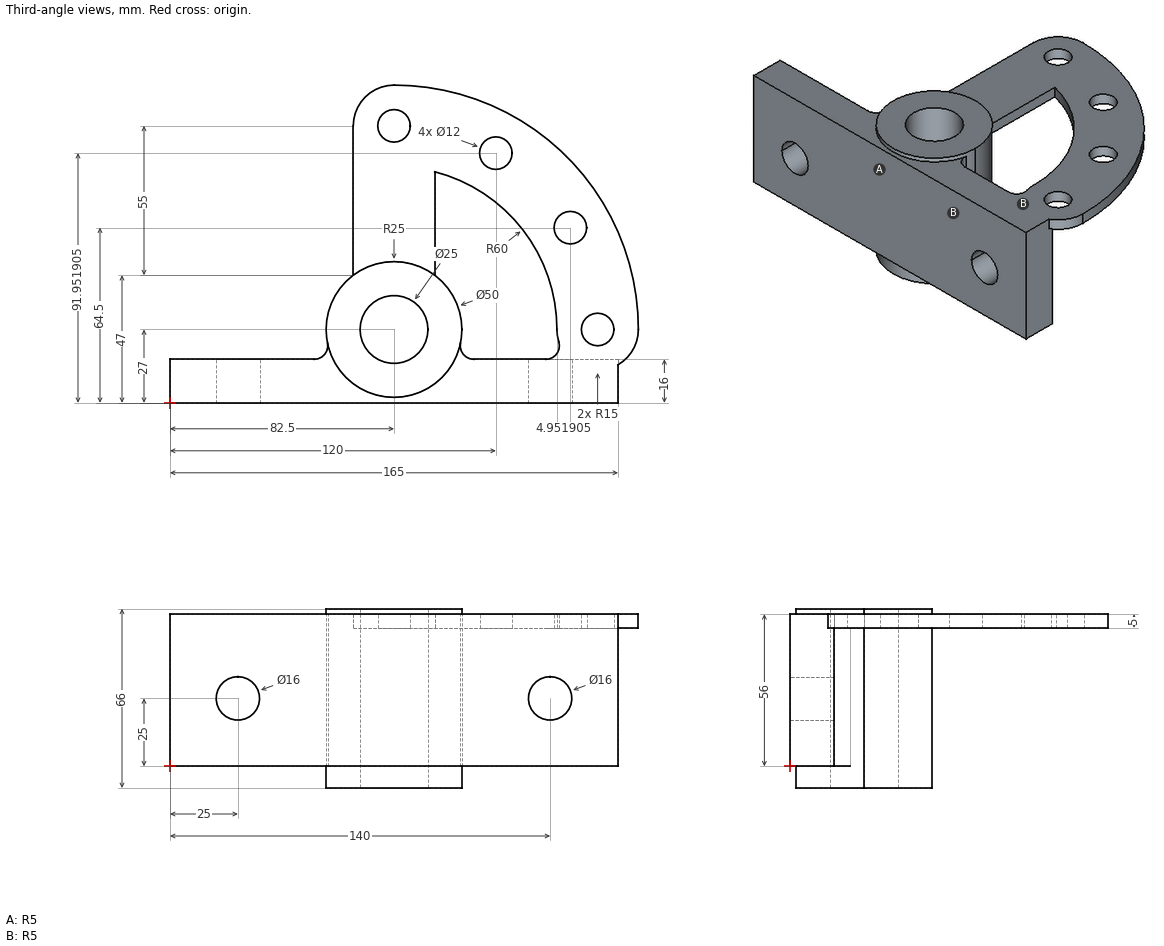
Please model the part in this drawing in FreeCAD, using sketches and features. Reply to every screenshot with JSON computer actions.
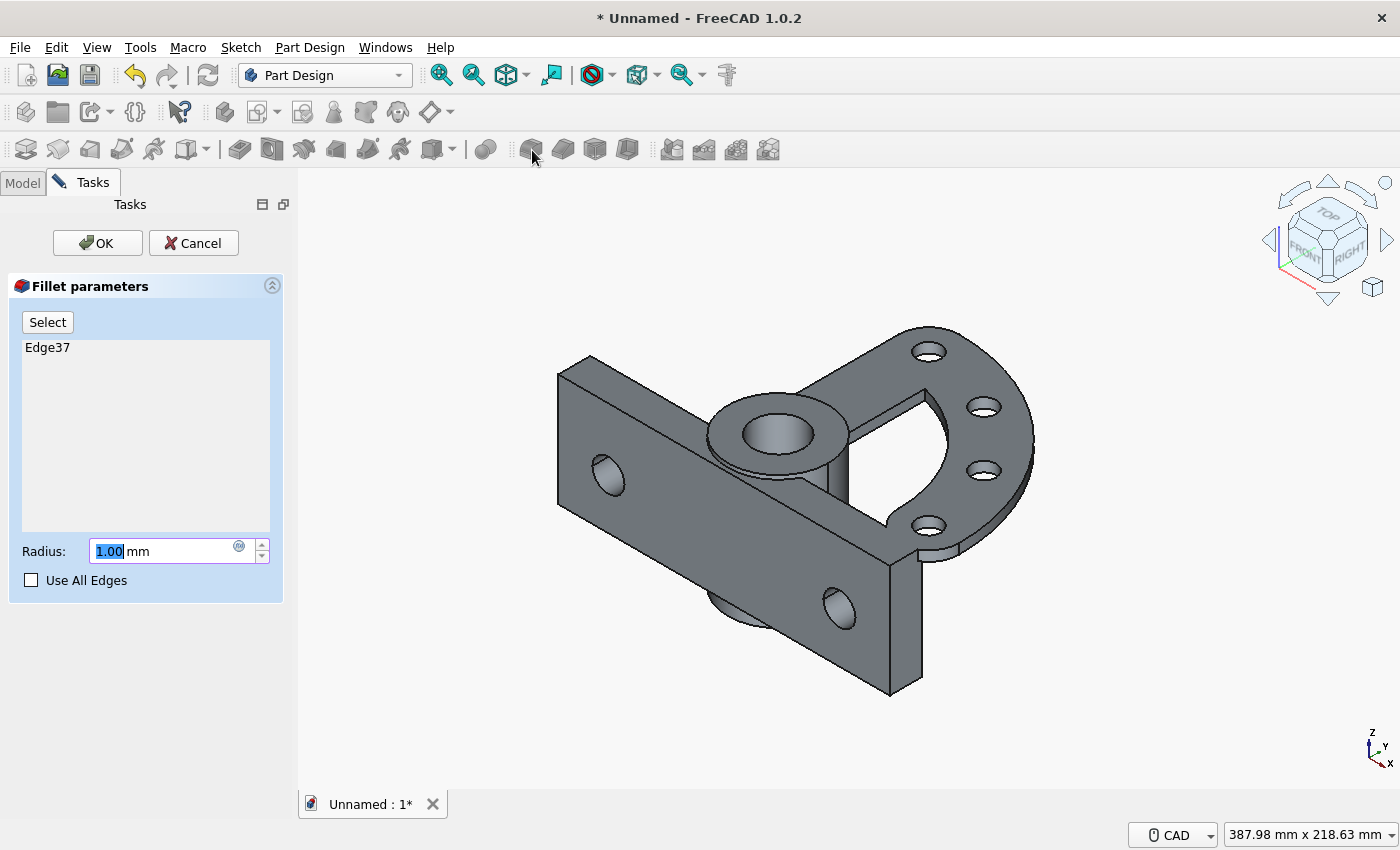
{"action": "type", "text": "5"}
{"action": "key", "text": "Tab"}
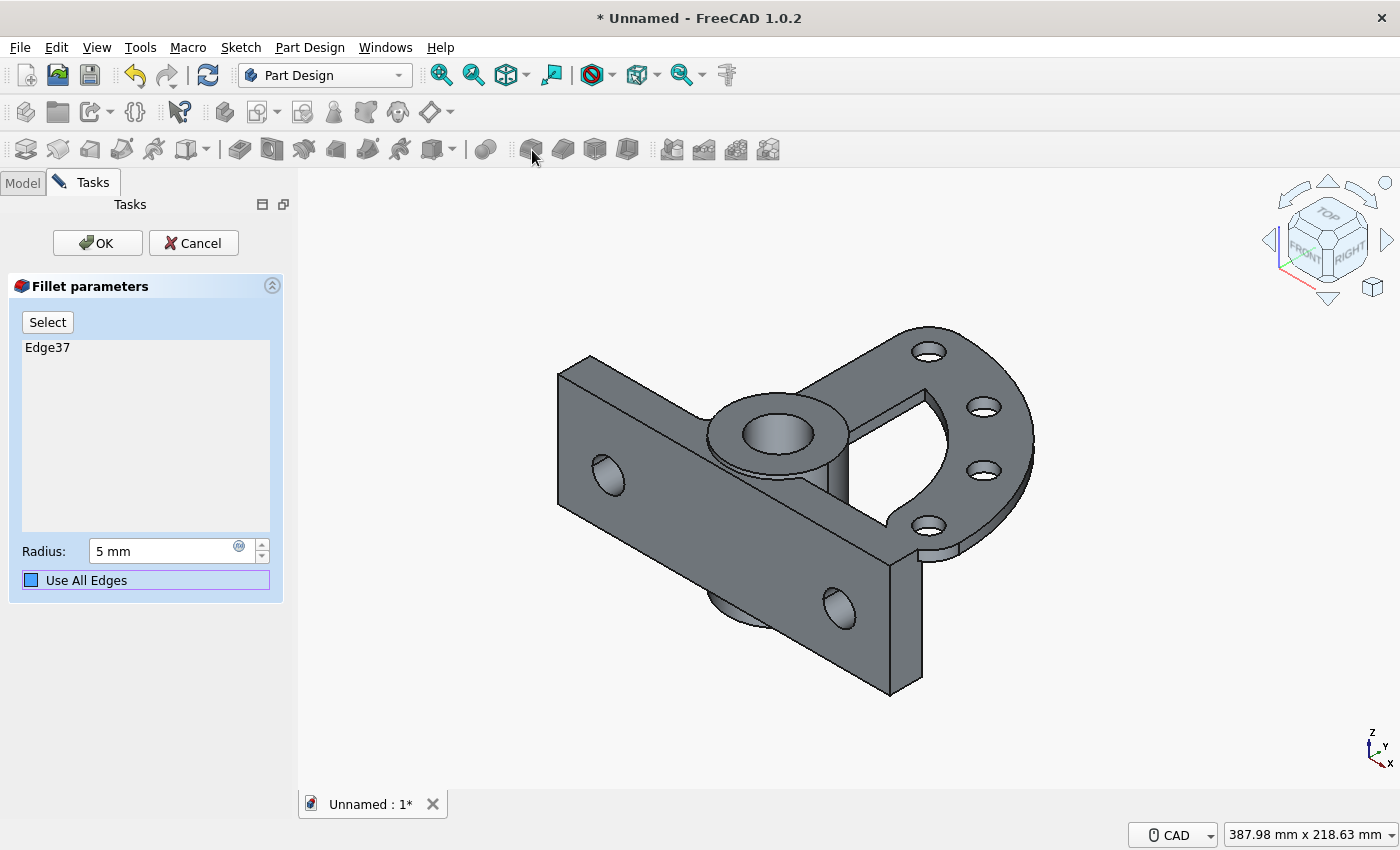
{"action": "left_click", "coordinate": [98, 243]}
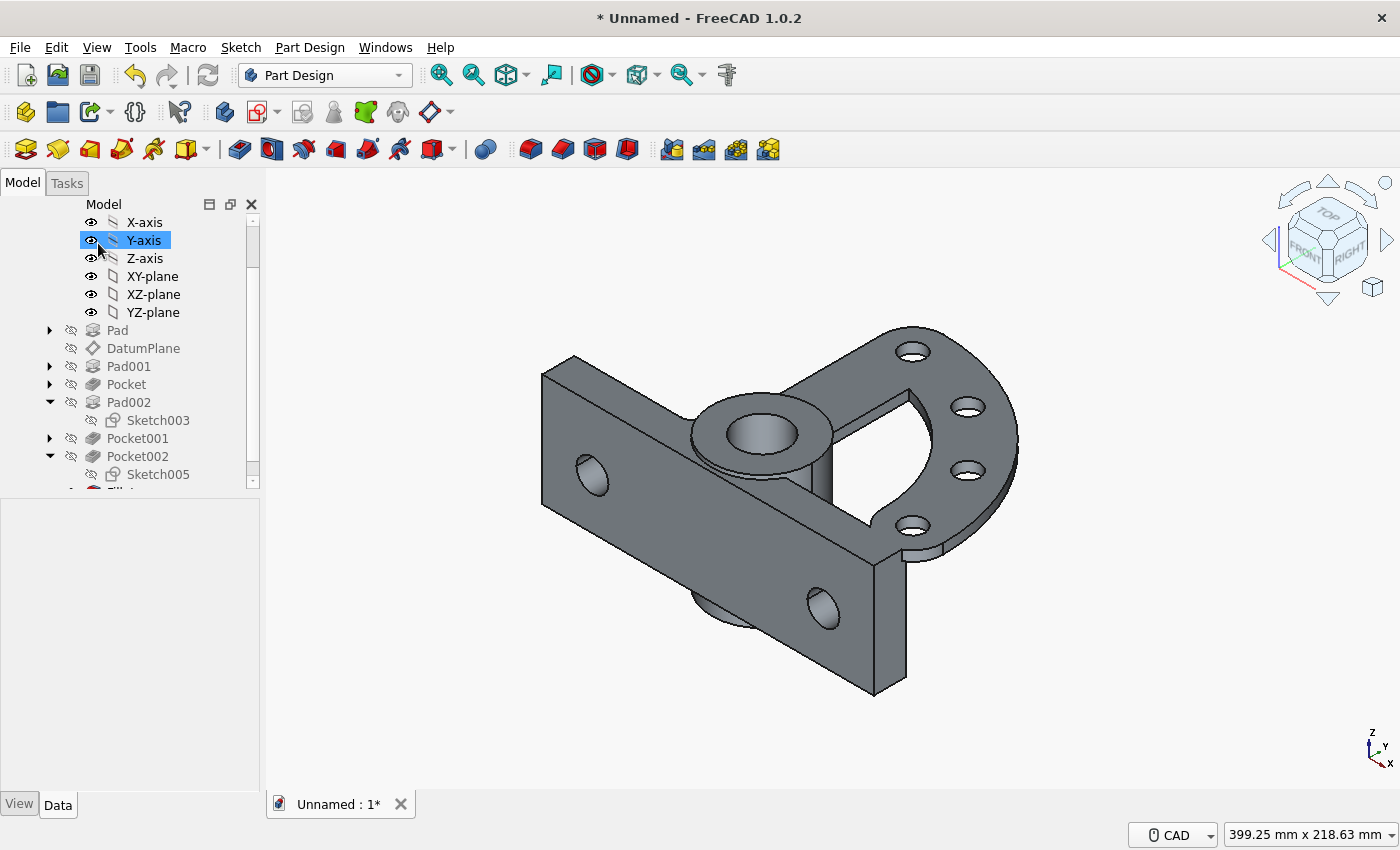
{"action": "key", "text": "2"}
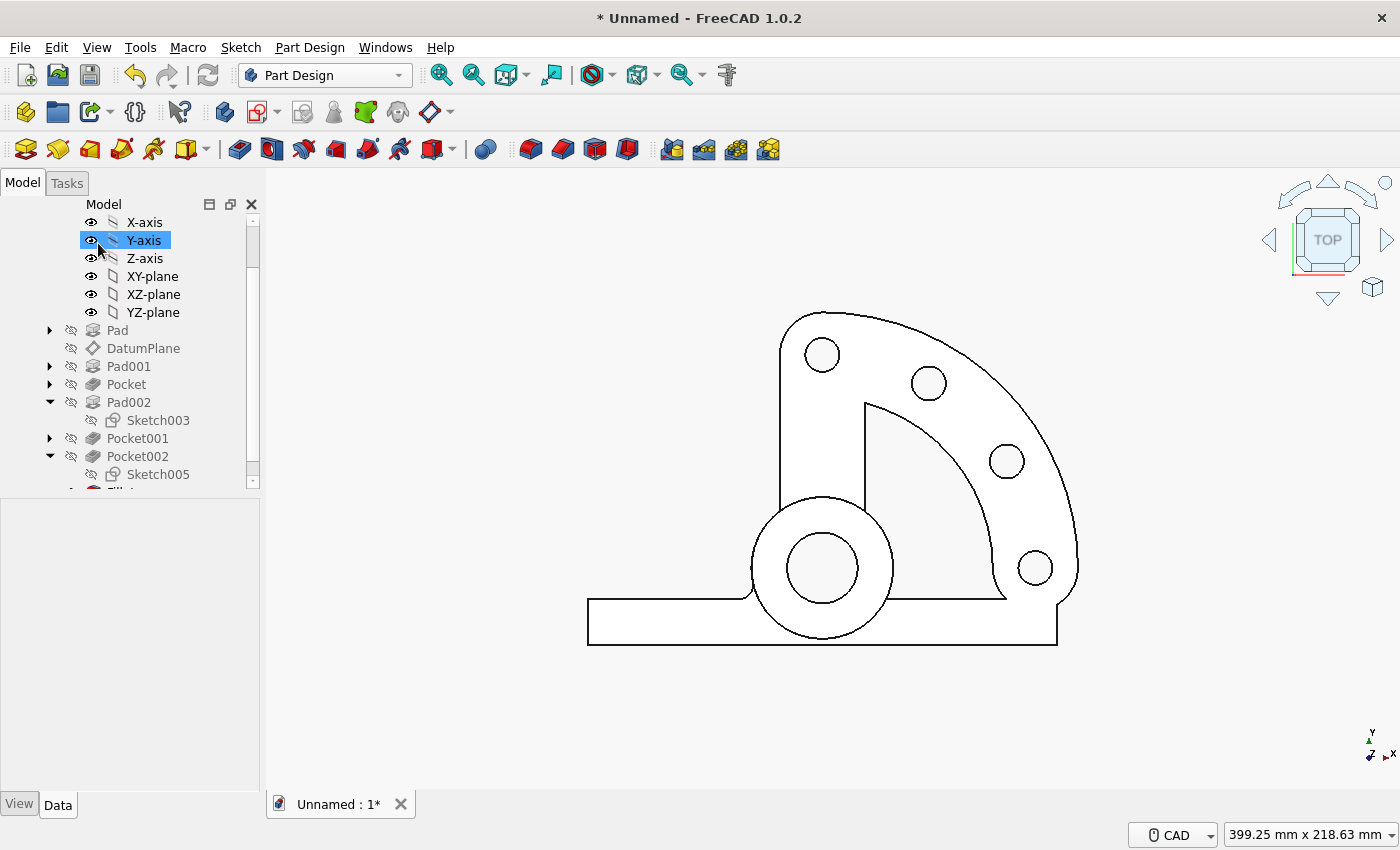
{"action": "key", "text": "0"}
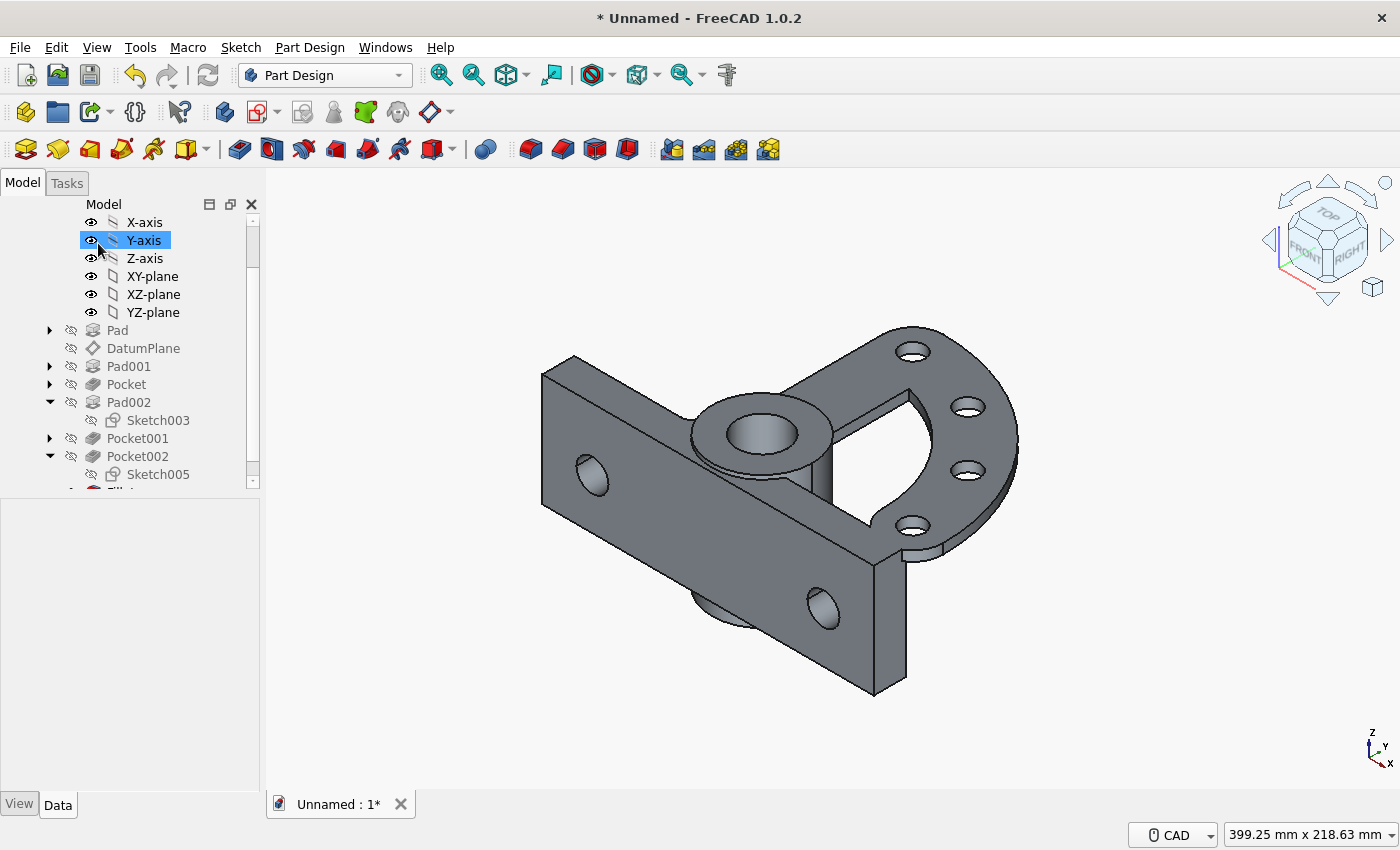
{"action": "key", "text": "1"}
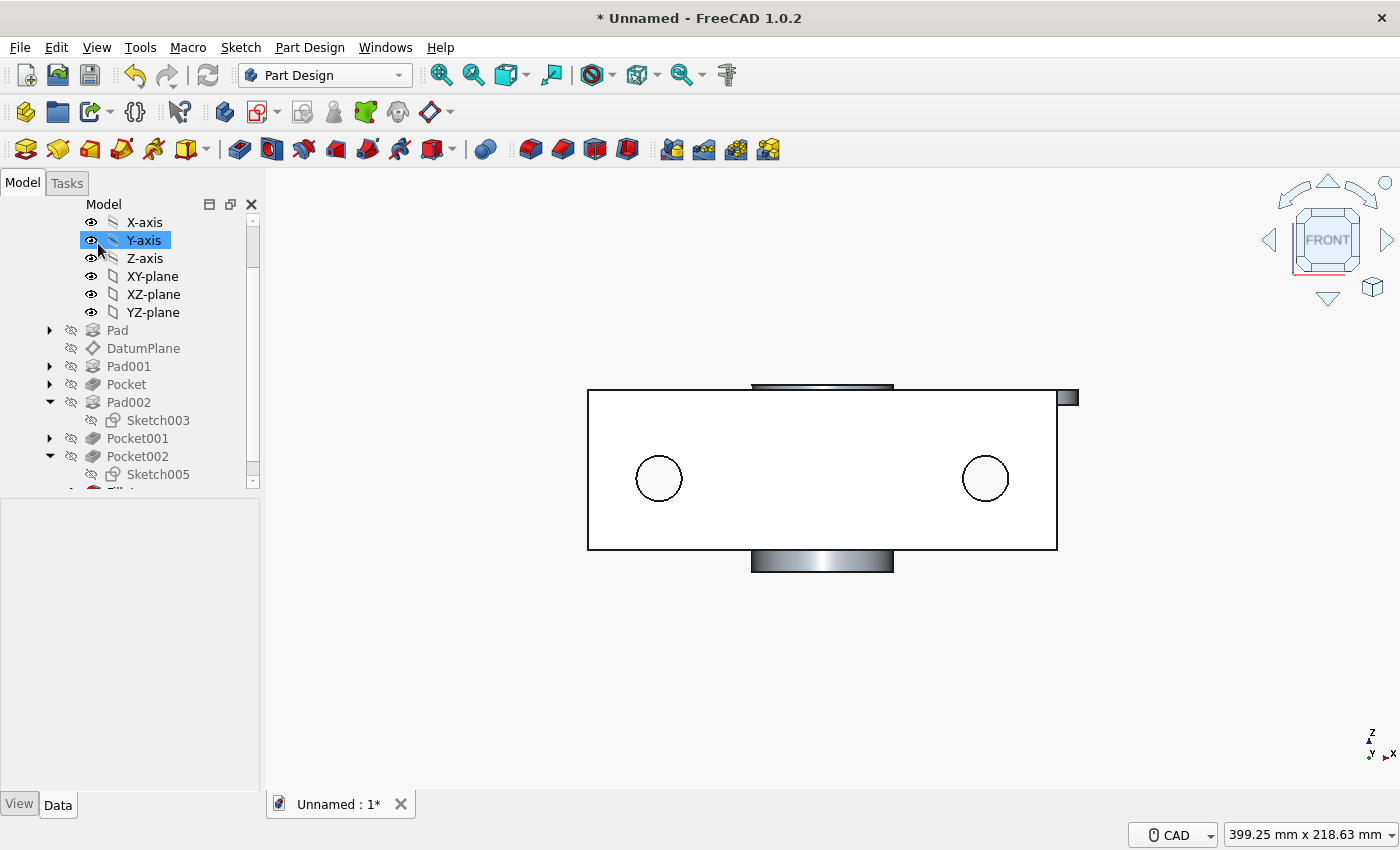
{"action": "key", "text": "v f"}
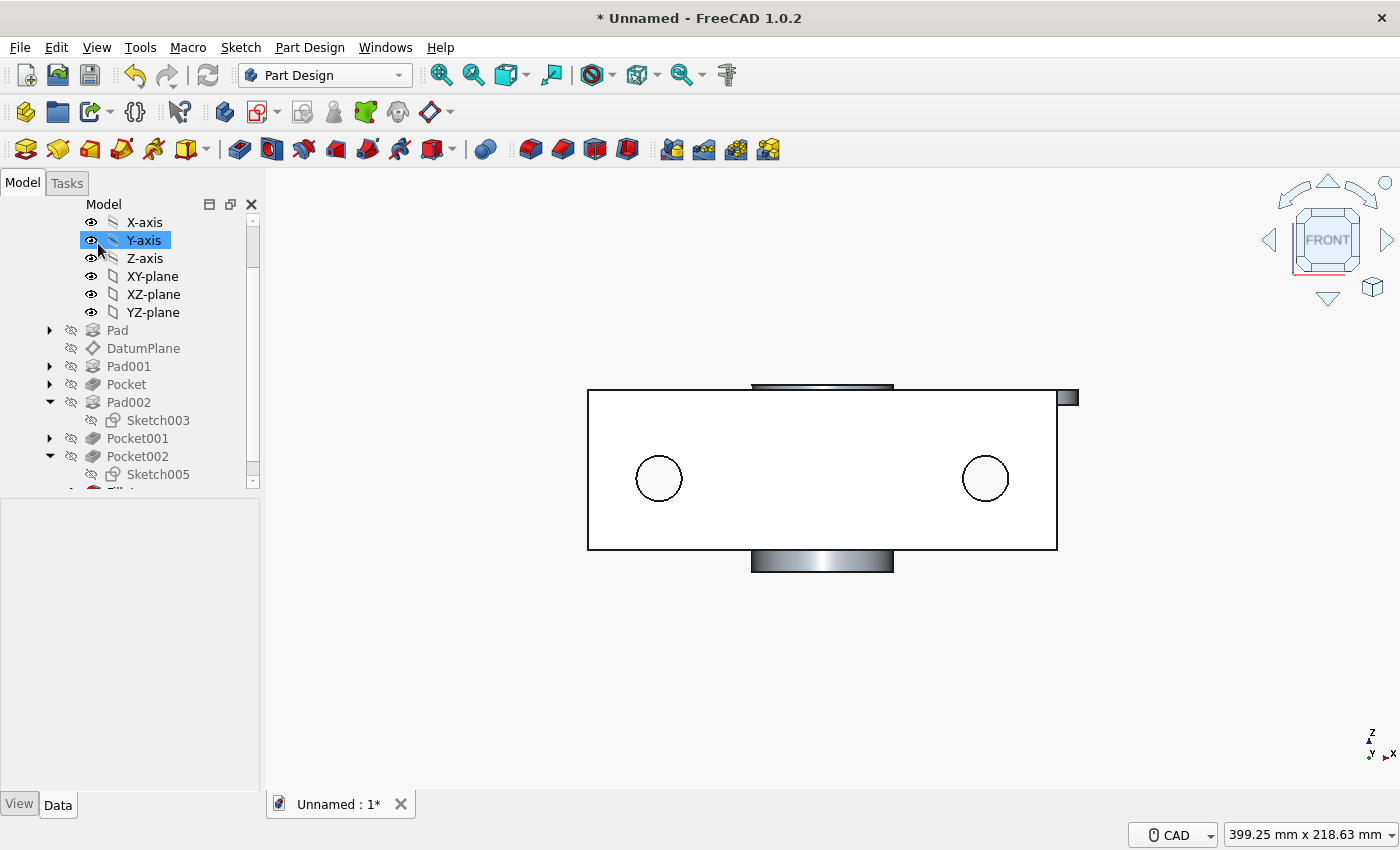
{"action": "key", "text": "3"}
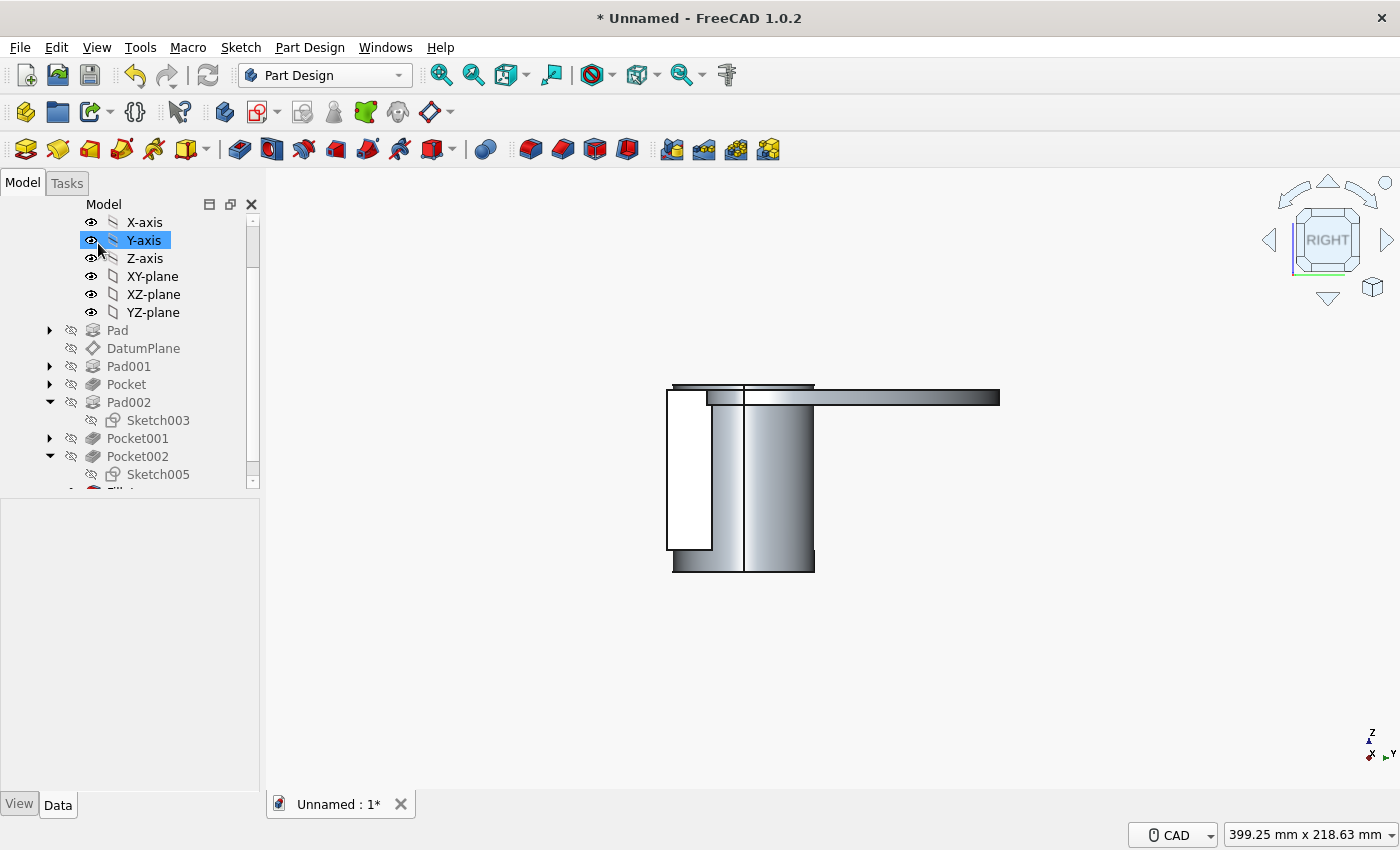
{"action": "key", "text": "v f"}